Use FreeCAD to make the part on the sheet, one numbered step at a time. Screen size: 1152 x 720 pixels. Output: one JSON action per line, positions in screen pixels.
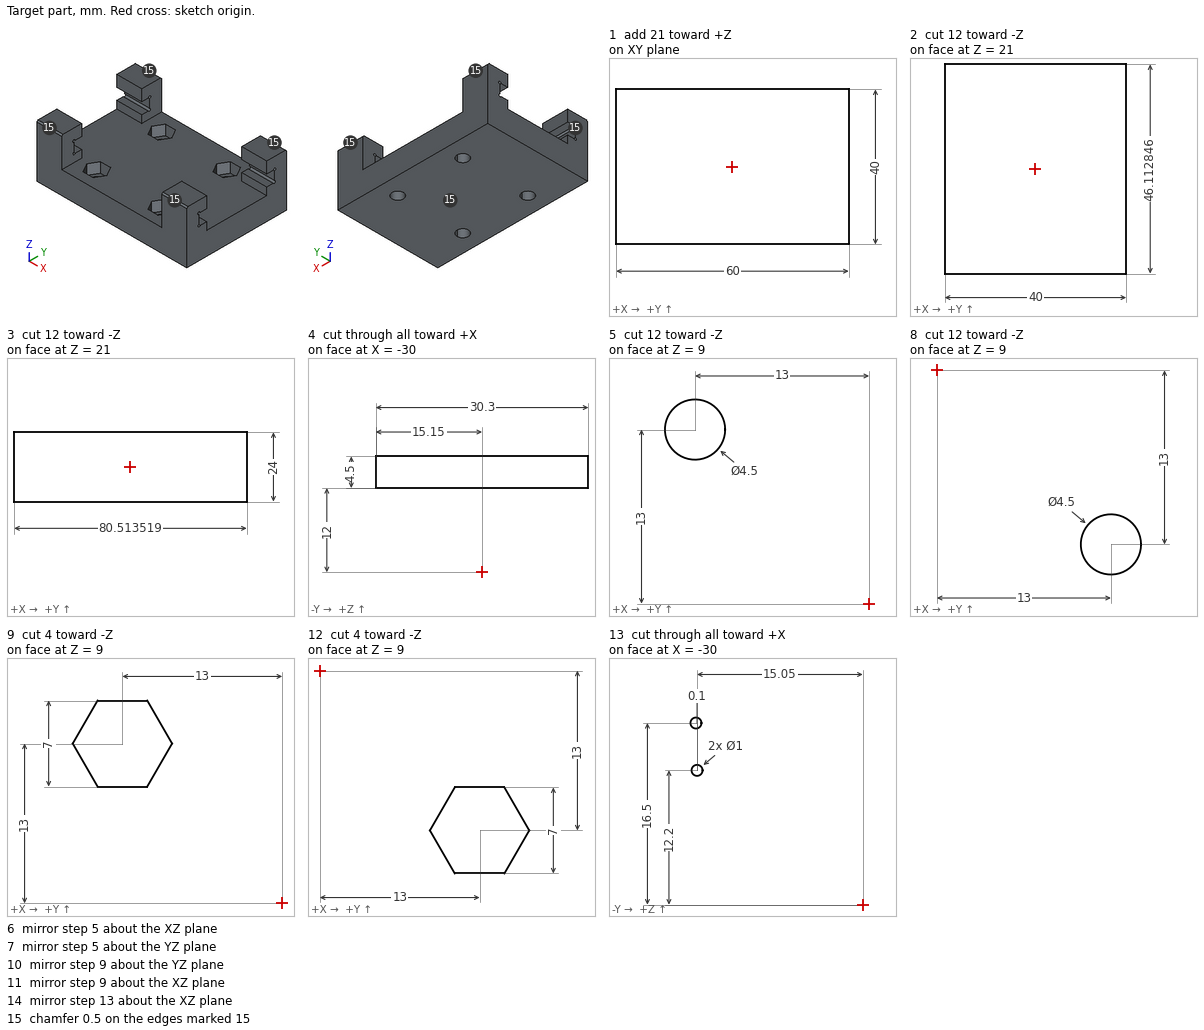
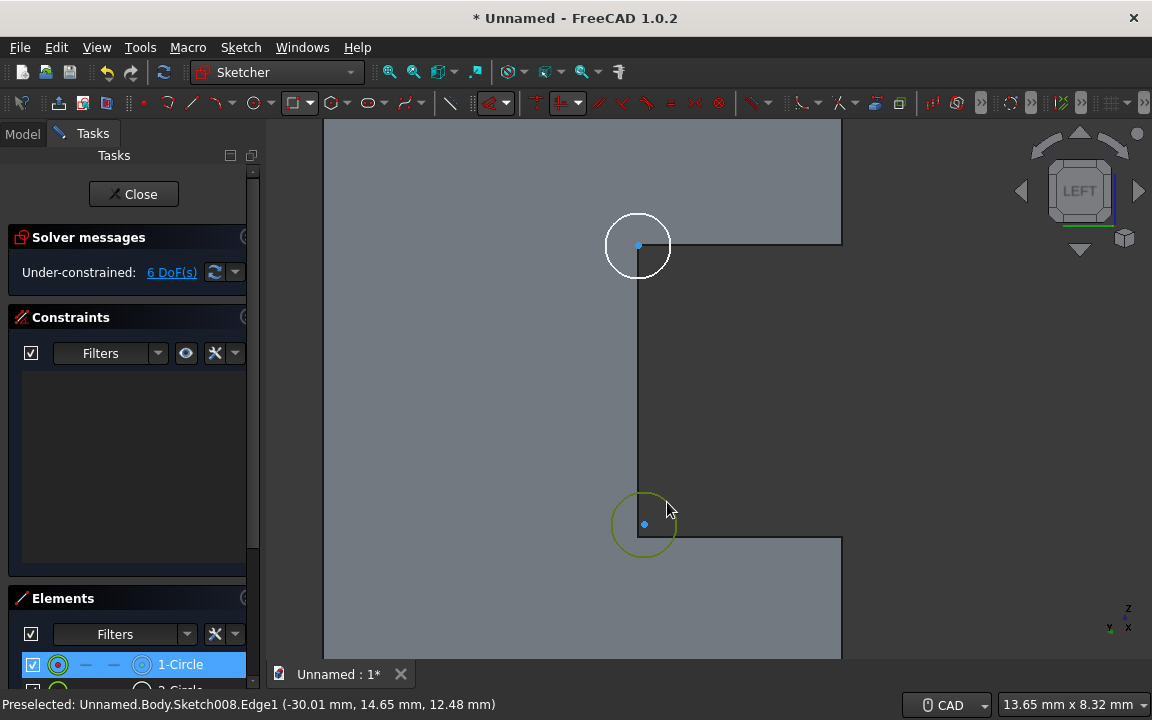
{"action": "left_click", "coordinate": [661, 223]}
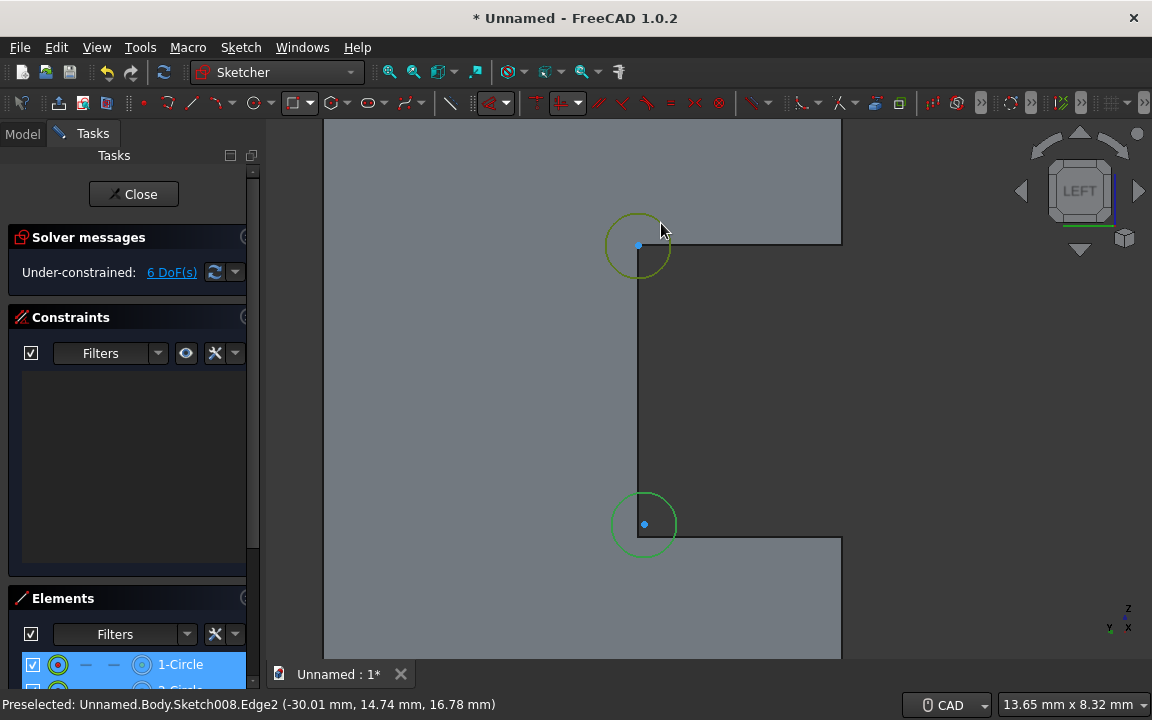
{"action": "left_click", "coordinate": [672, 104]}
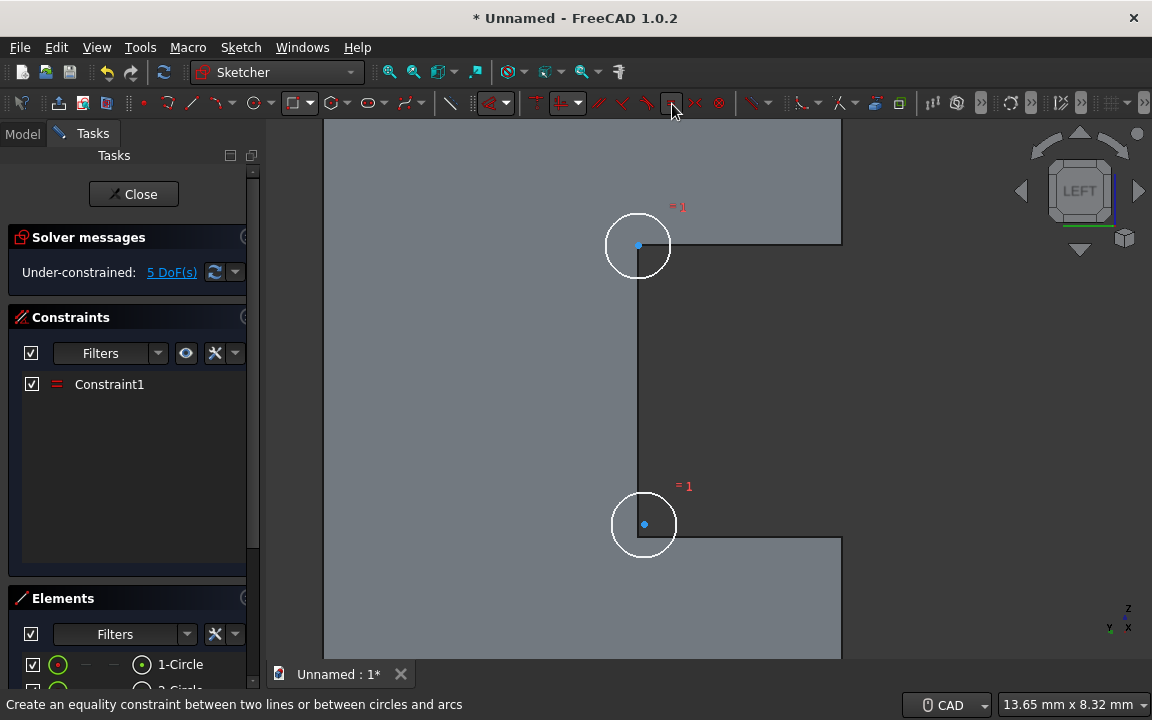
{"action": "left_click", "coordinate": [667, 502]}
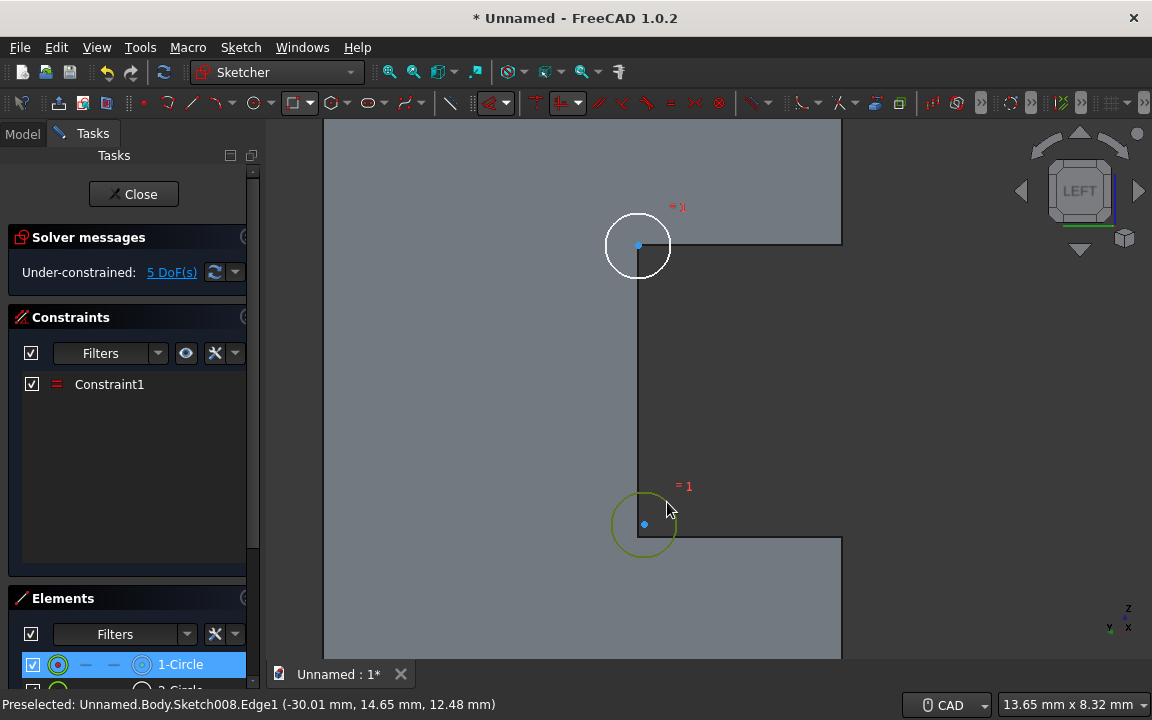
{"action": "key", "text": "k o"}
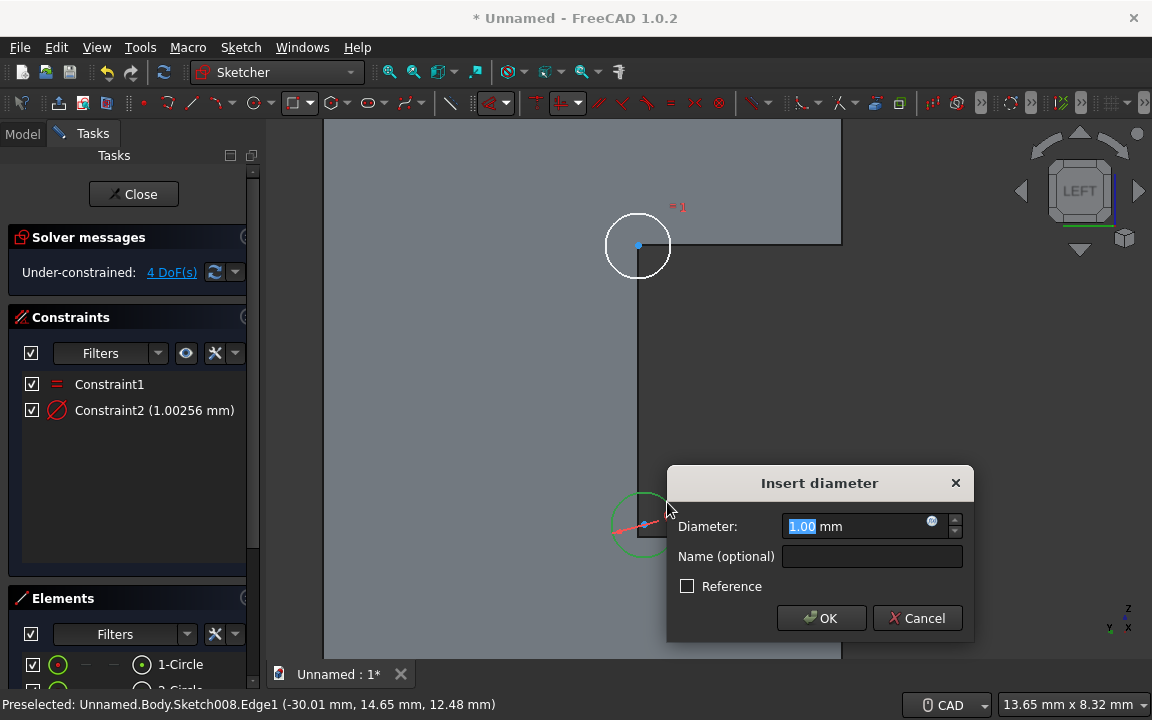
{"action": "type", "text": "1"}
{"action": "key", "text": "Return"}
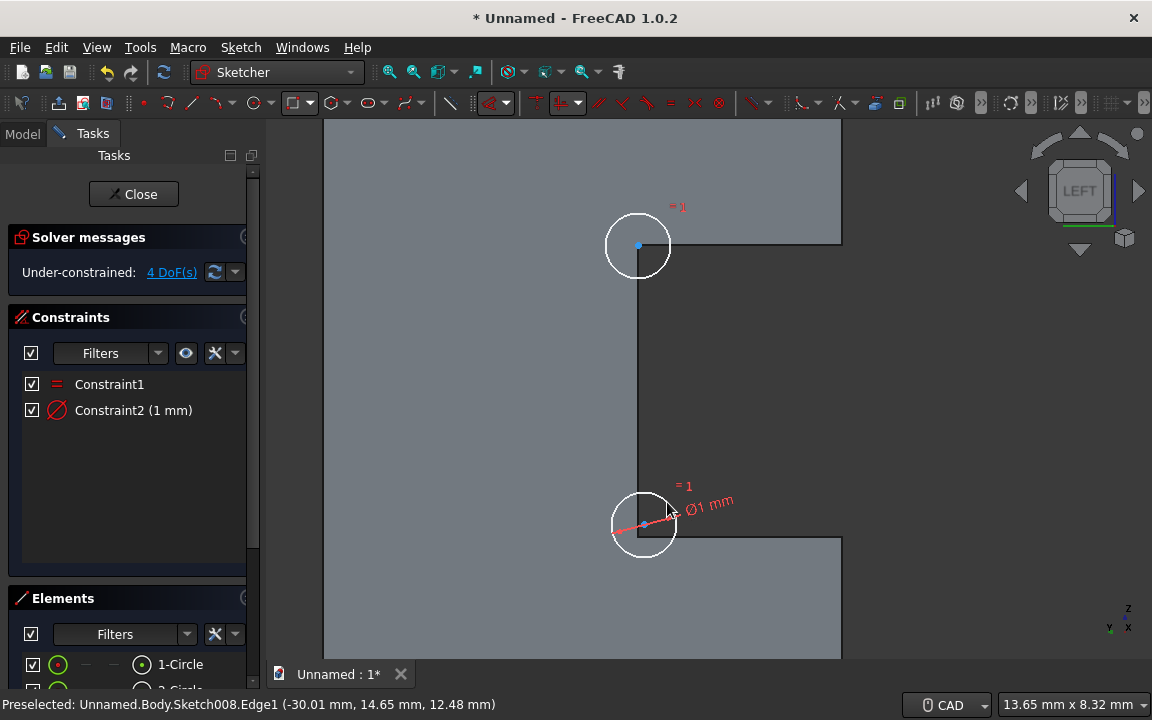
{"action": "left_click", "coordinate": [644, 525]}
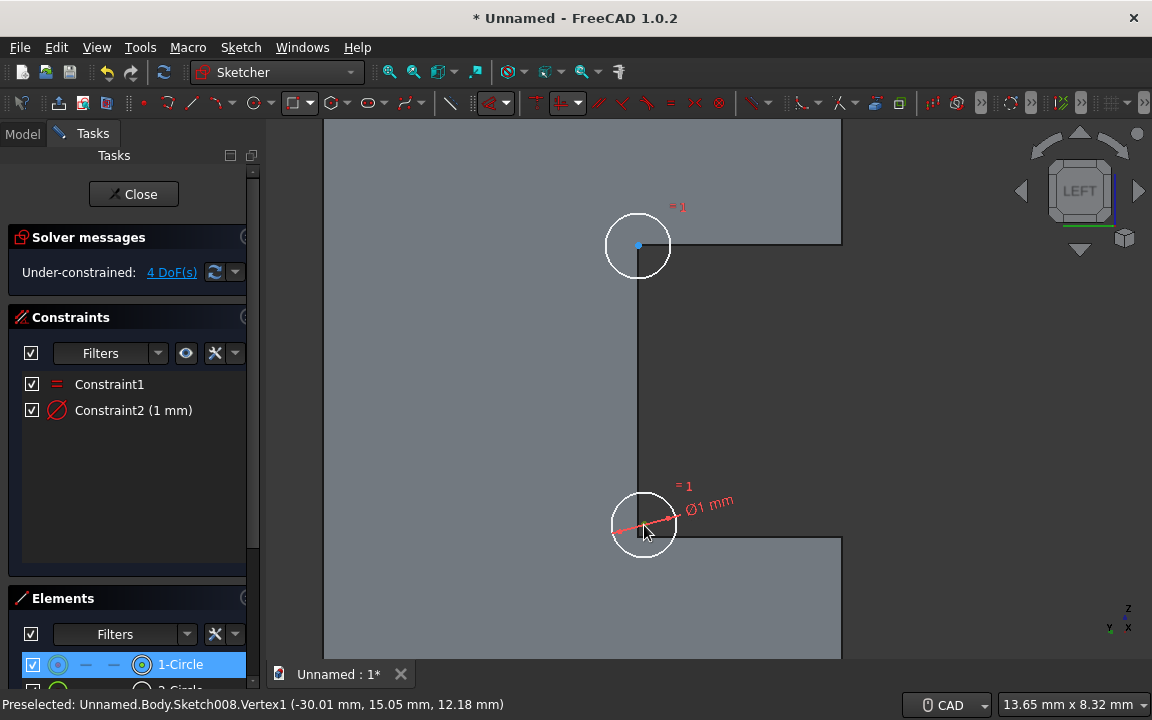
{"action": "left_click", "coordinate": [508, 104]}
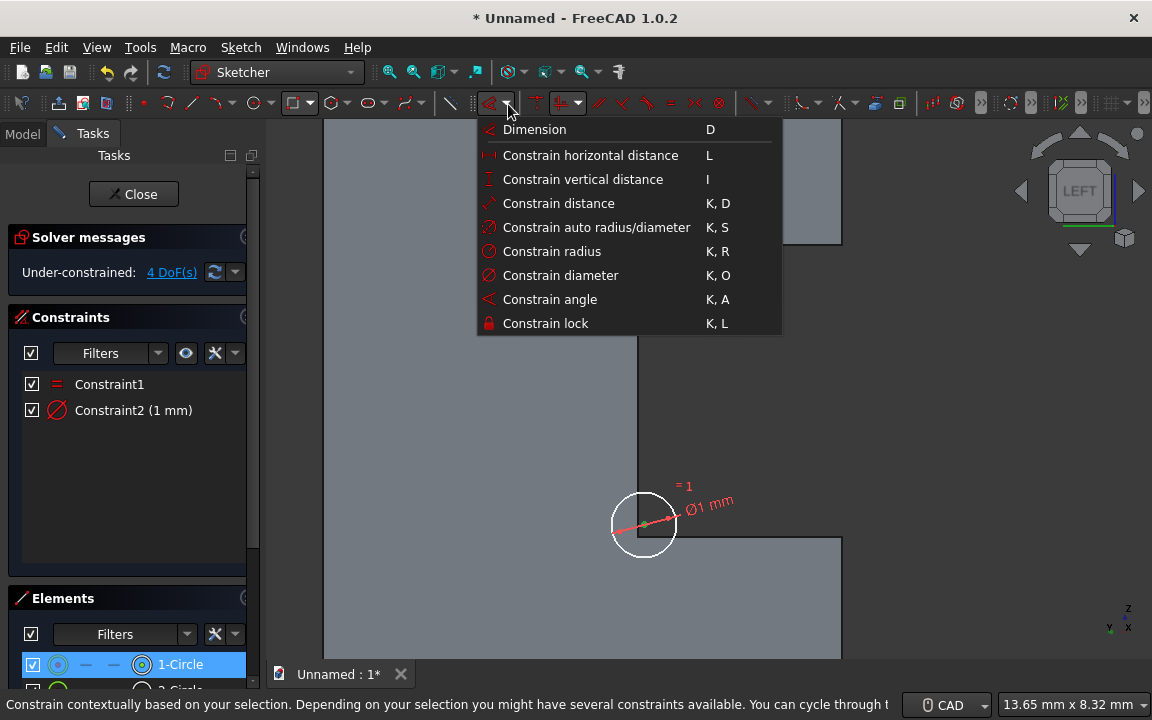
{"action": "left_click", "coordinate": [630, 179]}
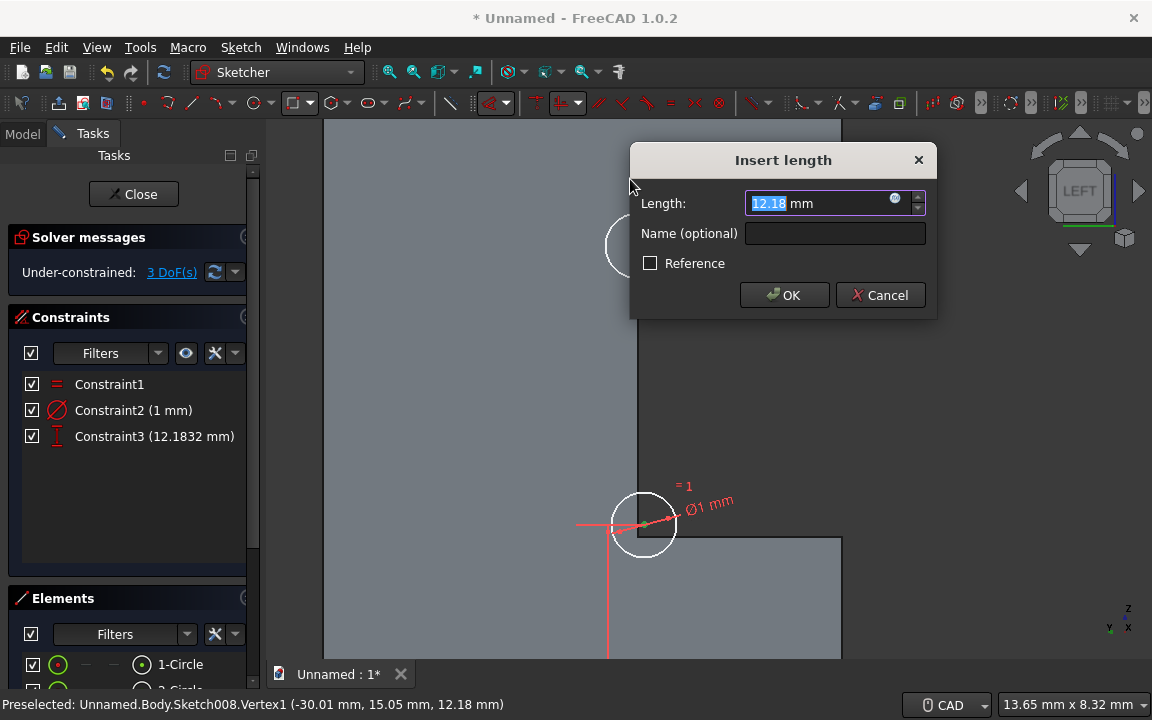
{"action": "type", "text": "12.2"}
{"action": "key", "text": "Return"}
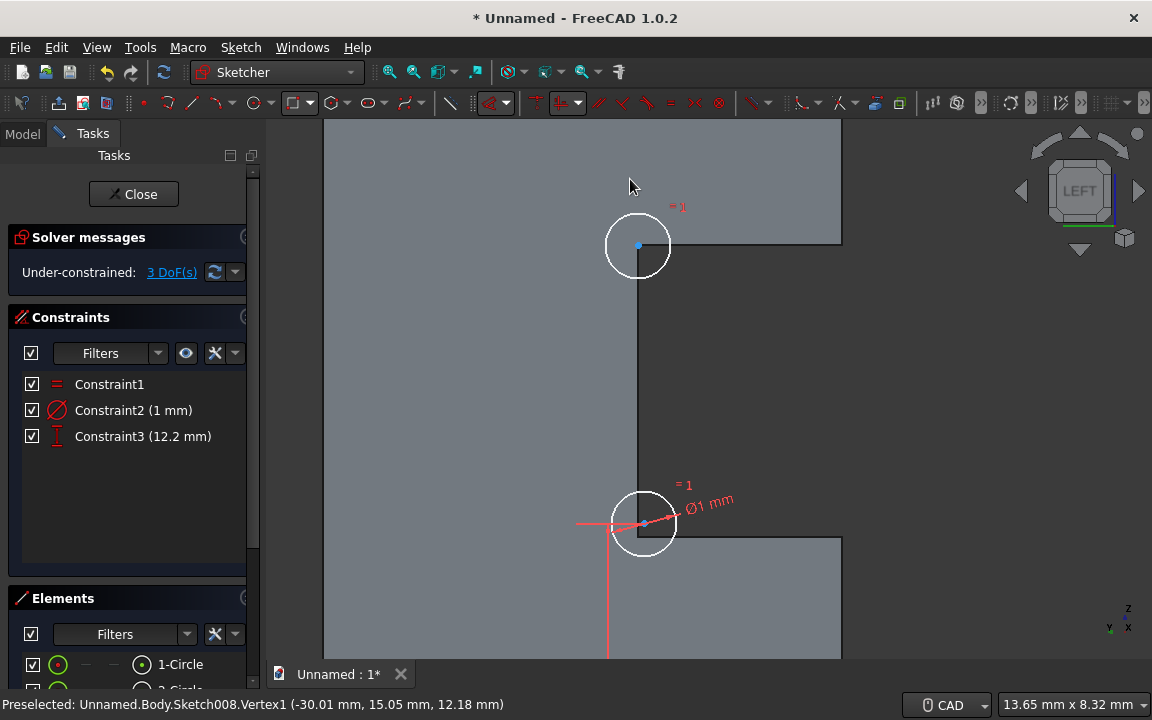
{"action": "left_click", "coordinate": [638, 246]}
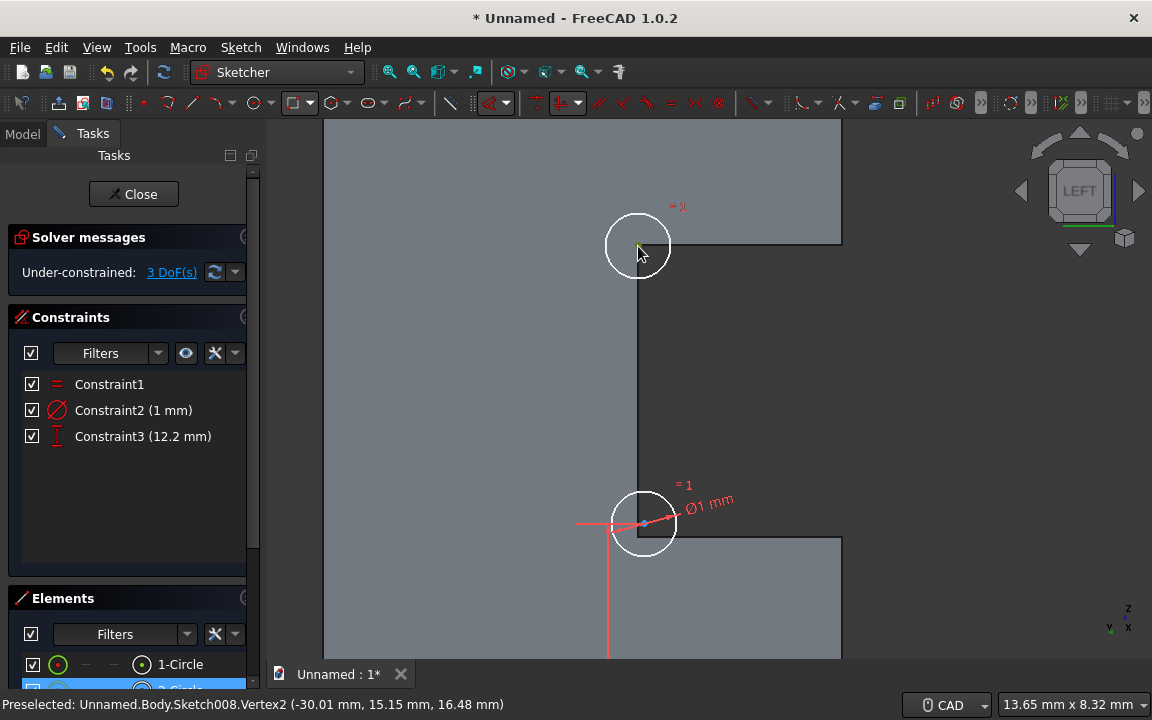
{"action": "key", "text": "i"}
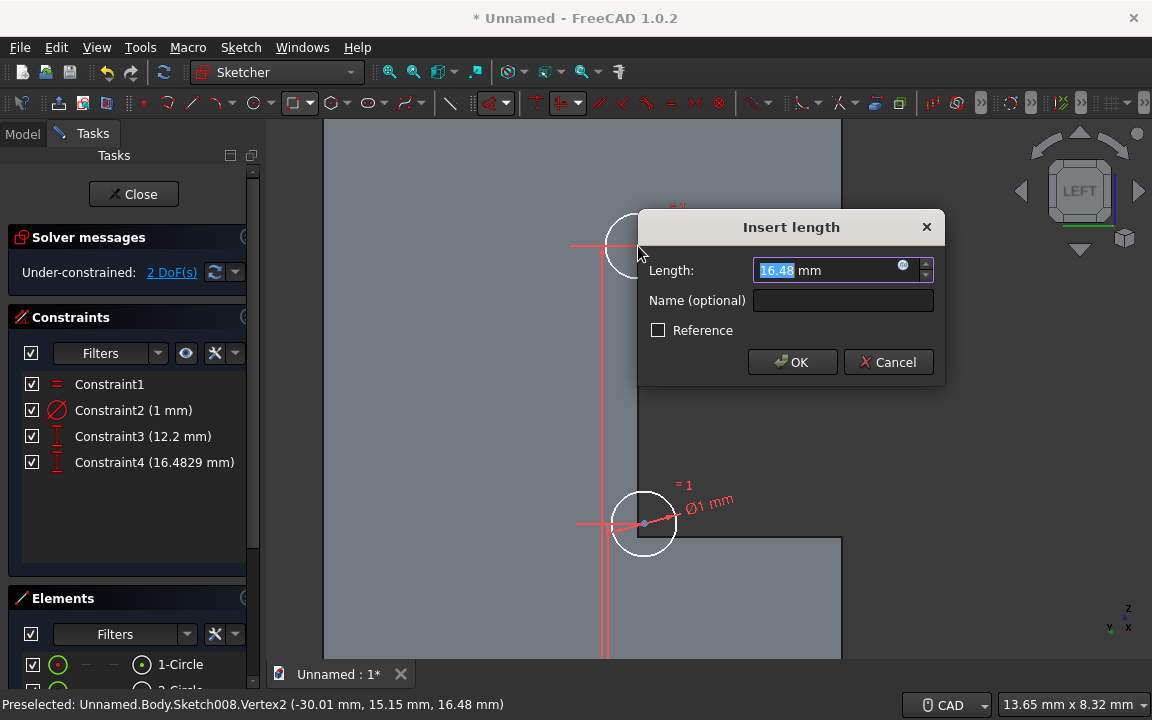
{"action": "type", "text": "16.5"}
{"action": "key", "text": "Return"}